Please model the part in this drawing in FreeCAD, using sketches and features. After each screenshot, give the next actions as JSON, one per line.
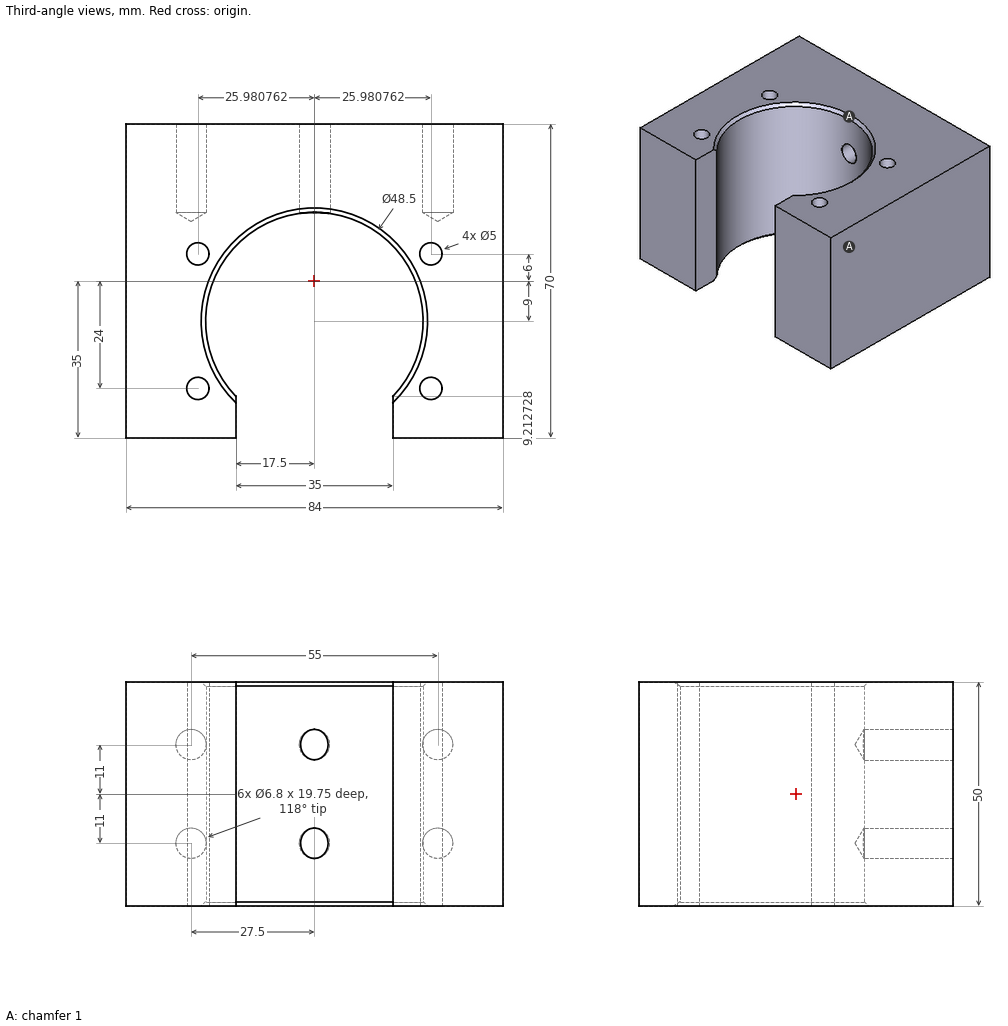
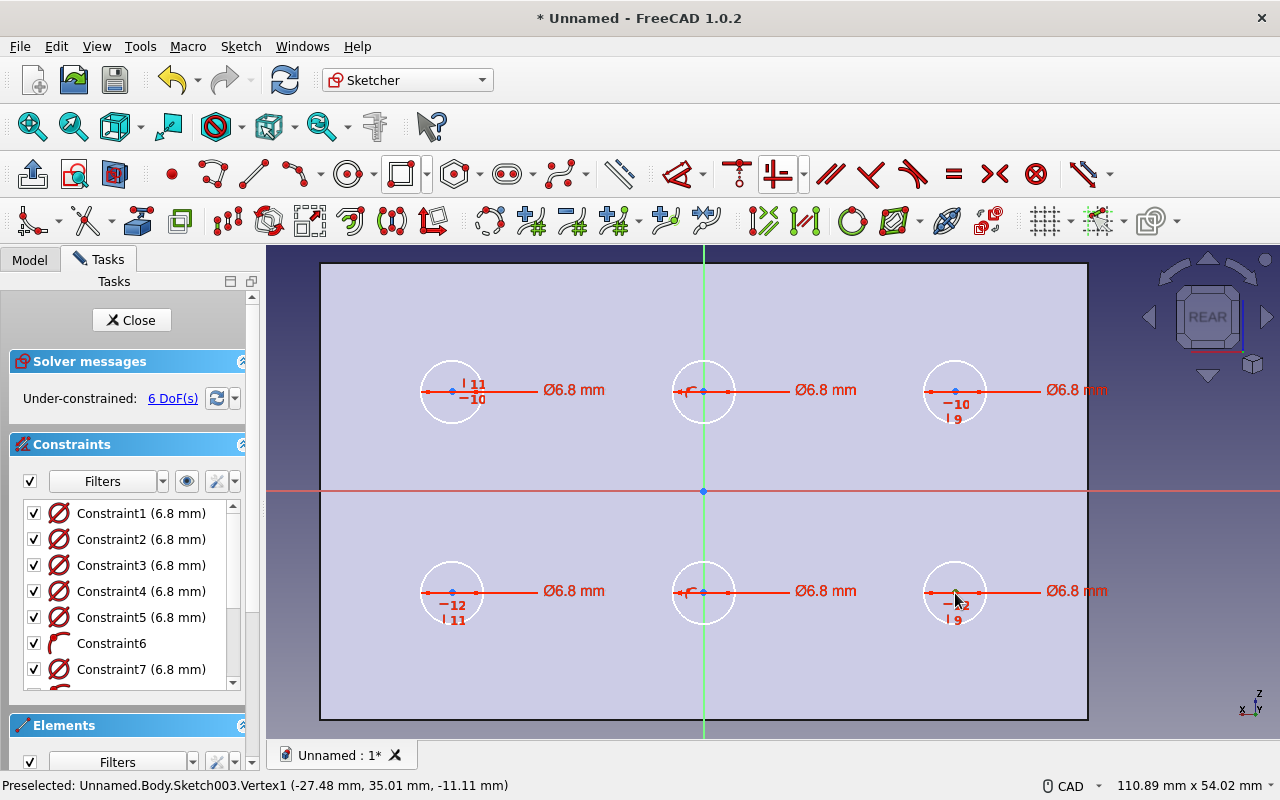
{"action": "left_click", "coordinate": [704, 593]}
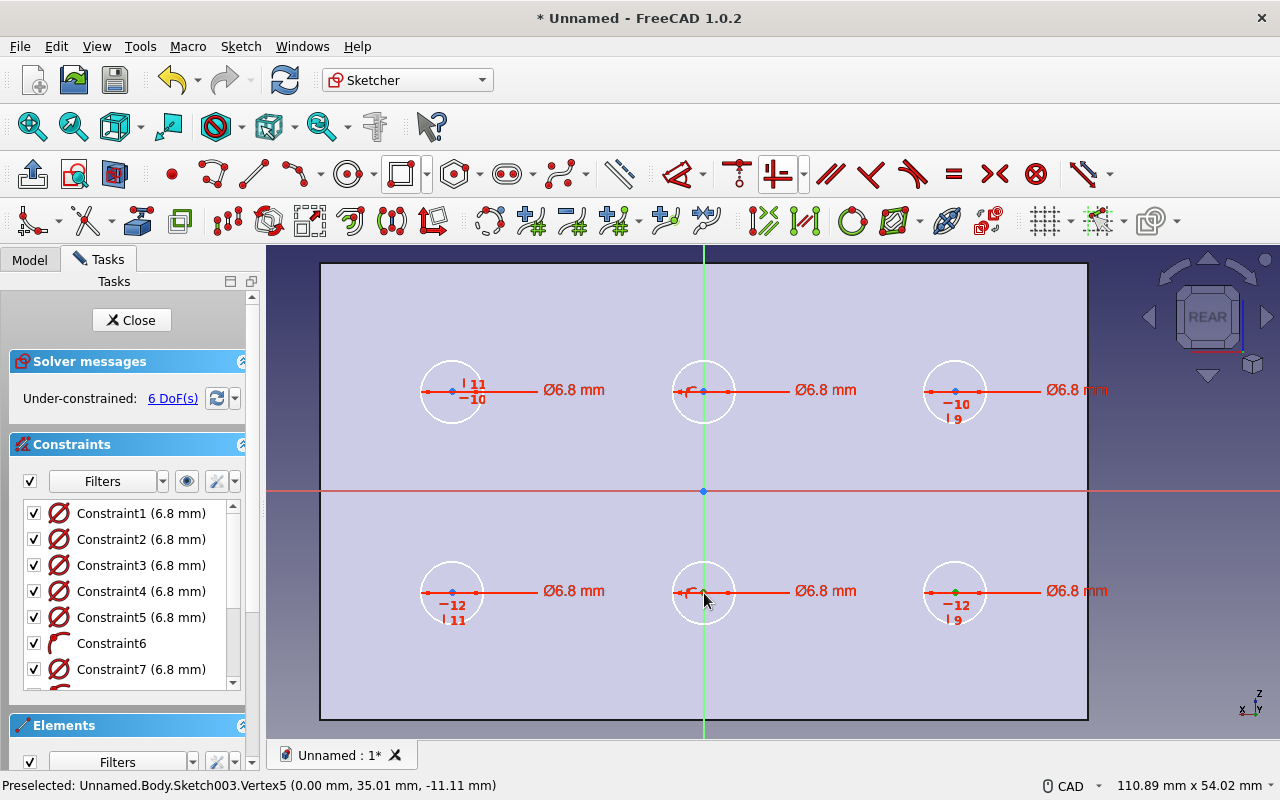
{"action": "key", "text": "h"}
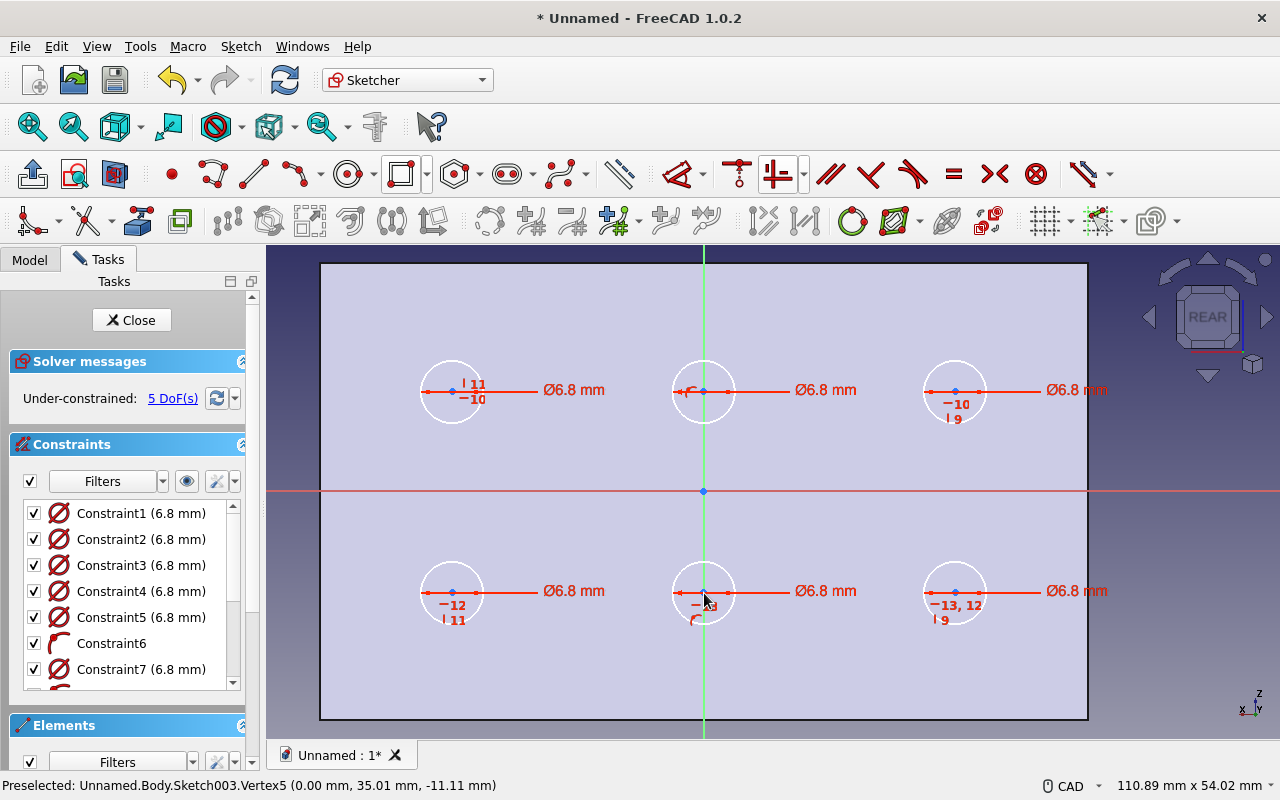
{"action": "left_click", "coordinate": [955, 392]}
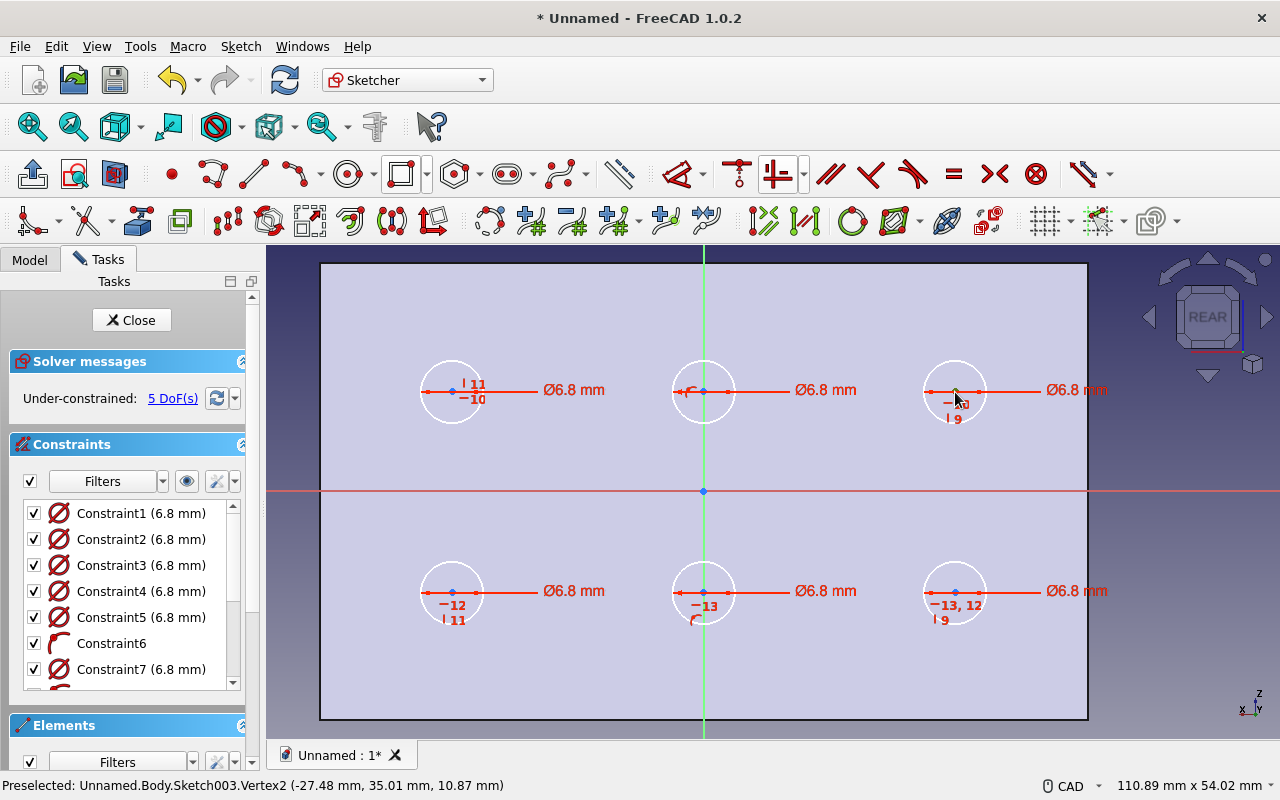
{"action": "left_click", "coordinate": [704, 392]}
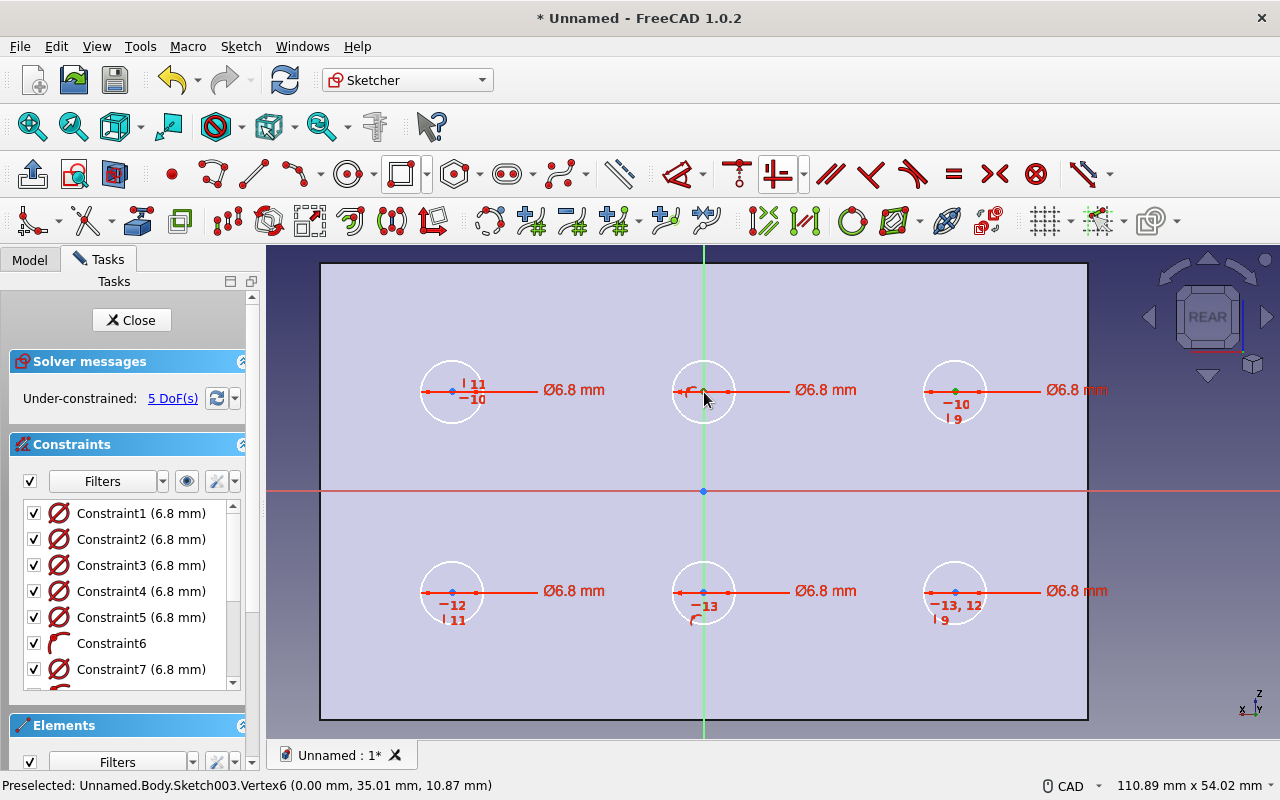
{"action": "key", "text": "h"}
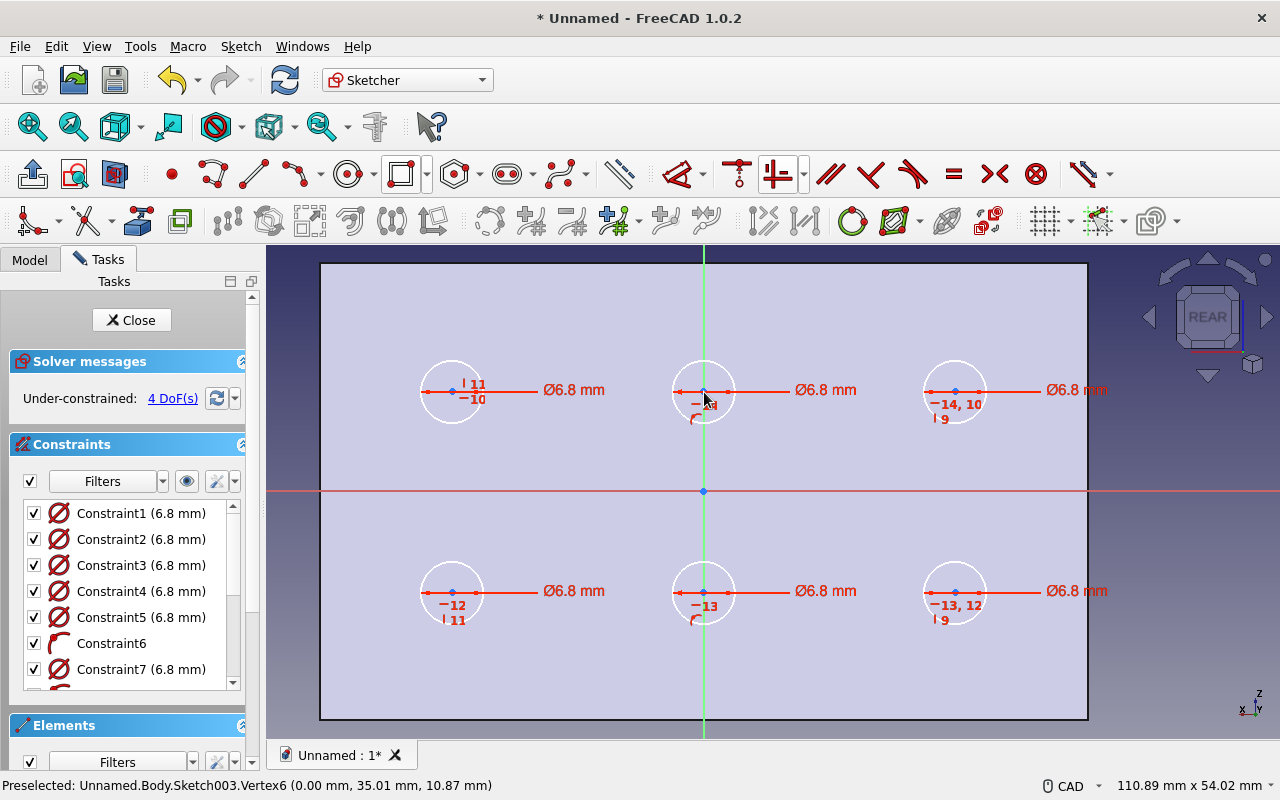
{"action": "key", "text": "d"}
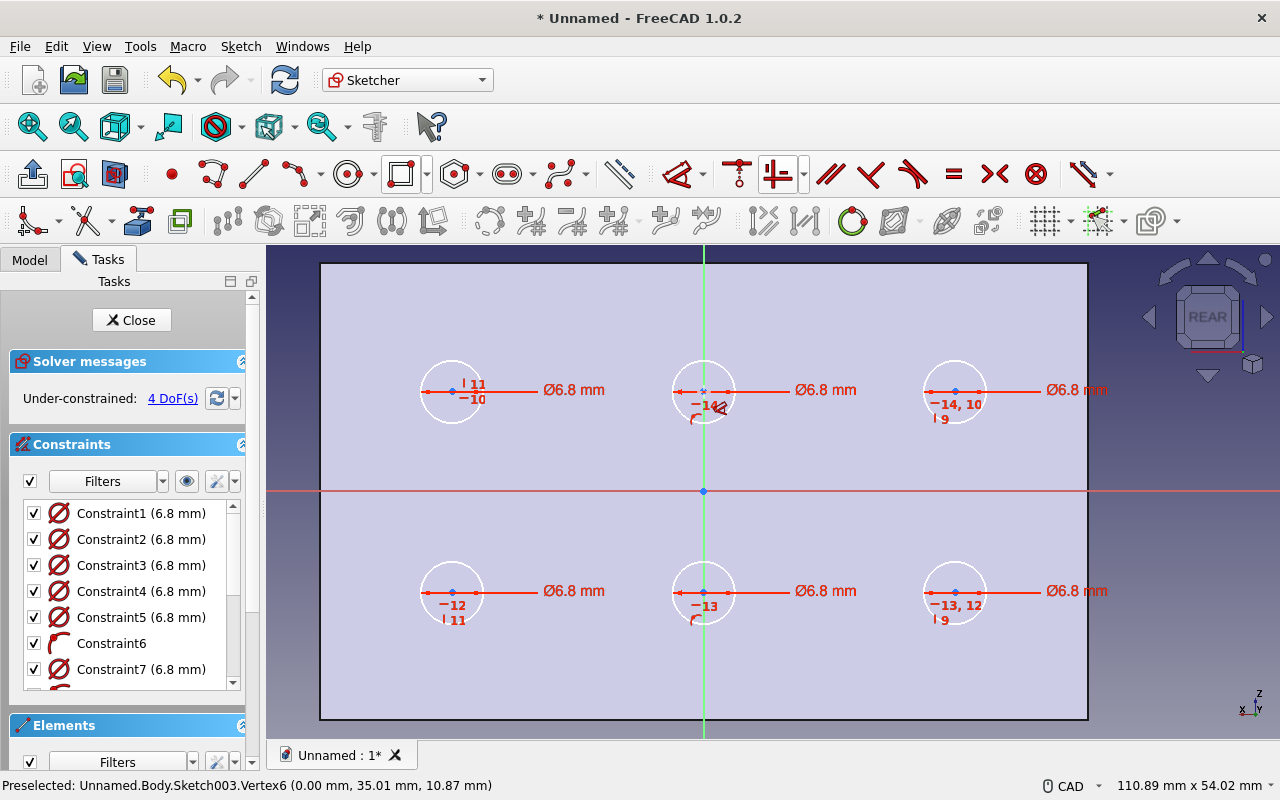
{"action": "left_click", "coordinate": [955, 593]}
{"action": "left_click", "coordinate": [989, 542]}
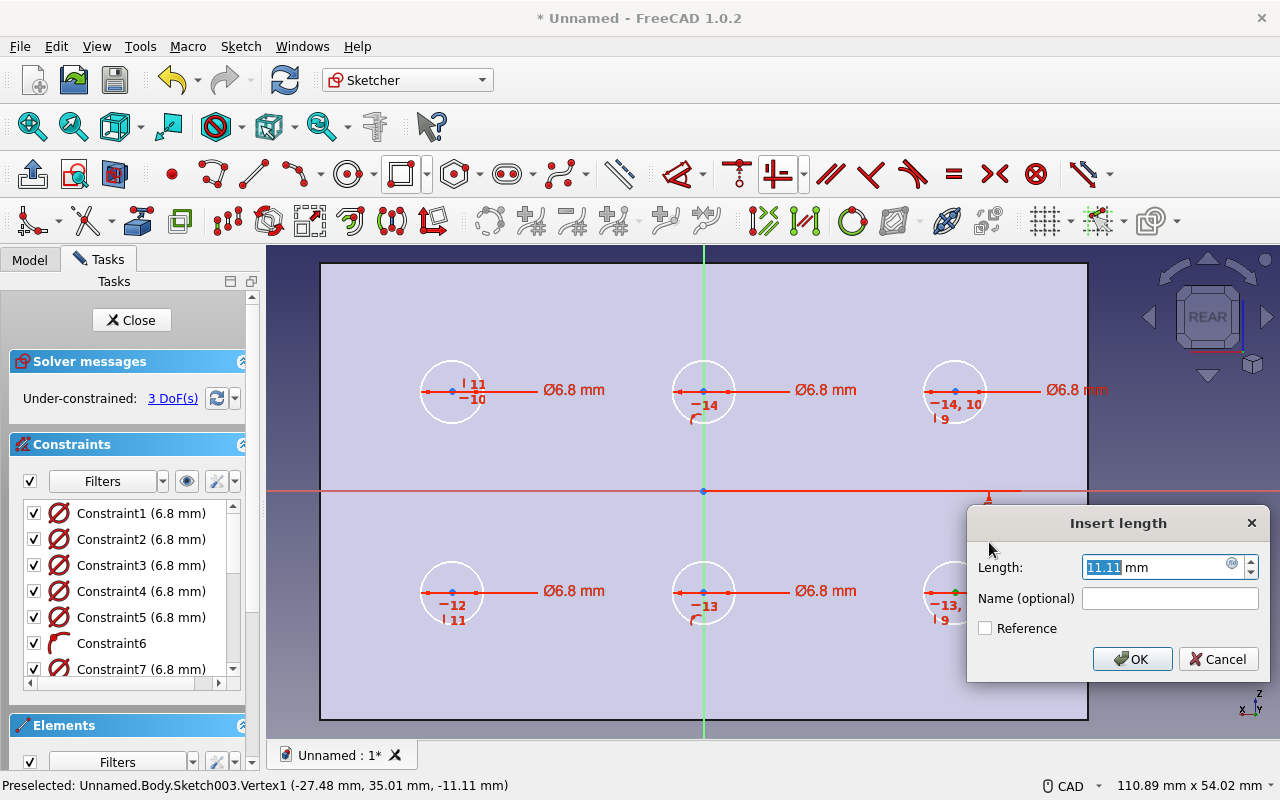
{"action": "type", "text": "11"}
{"action": "key", "text": "Return"}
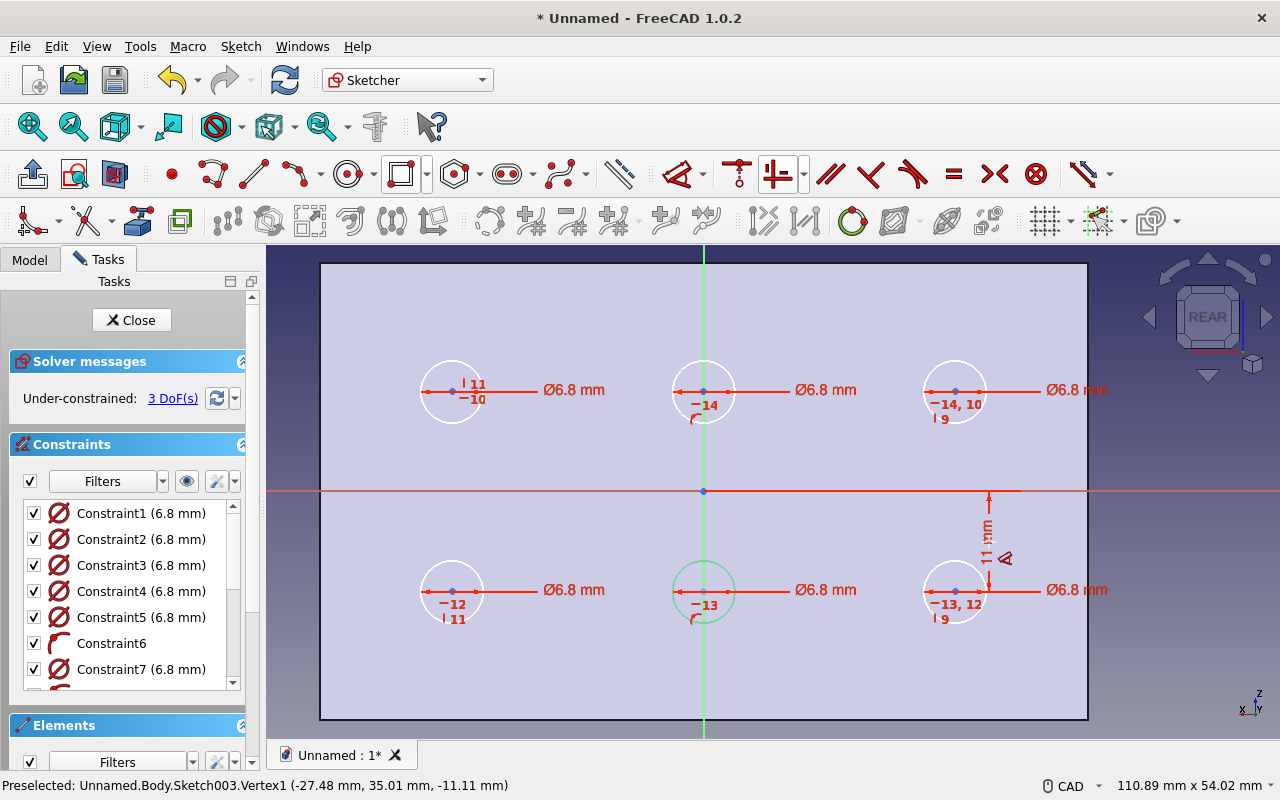
{"action": "left_click", "coordinate": [955, 392]}
{"action": "left_click", "coordinate": [989, 442]}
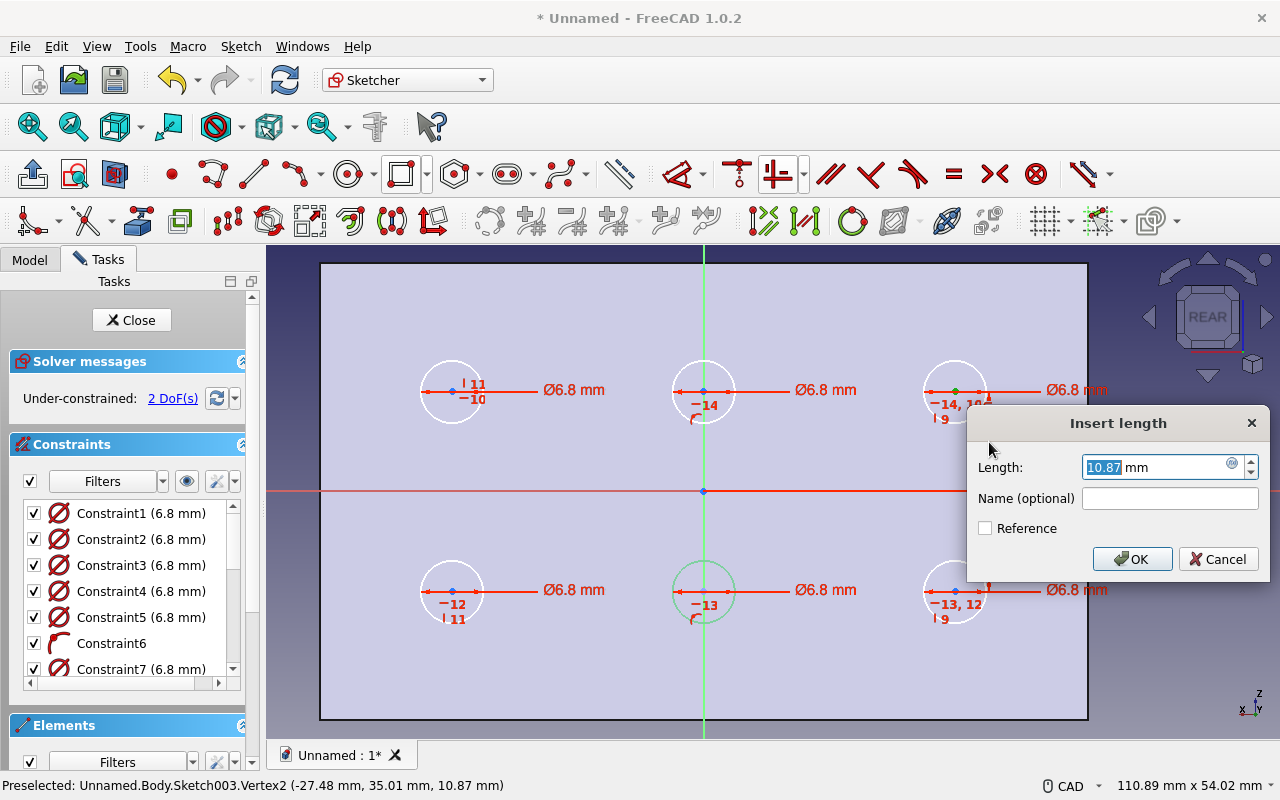
{"action": "type", "text": "11"}
{"action": "key", "text": "Return"}